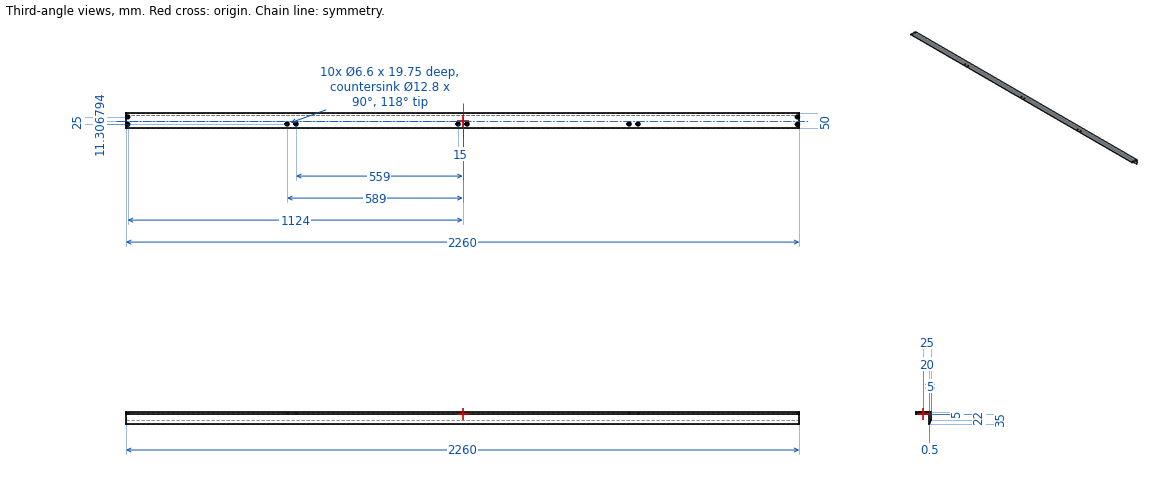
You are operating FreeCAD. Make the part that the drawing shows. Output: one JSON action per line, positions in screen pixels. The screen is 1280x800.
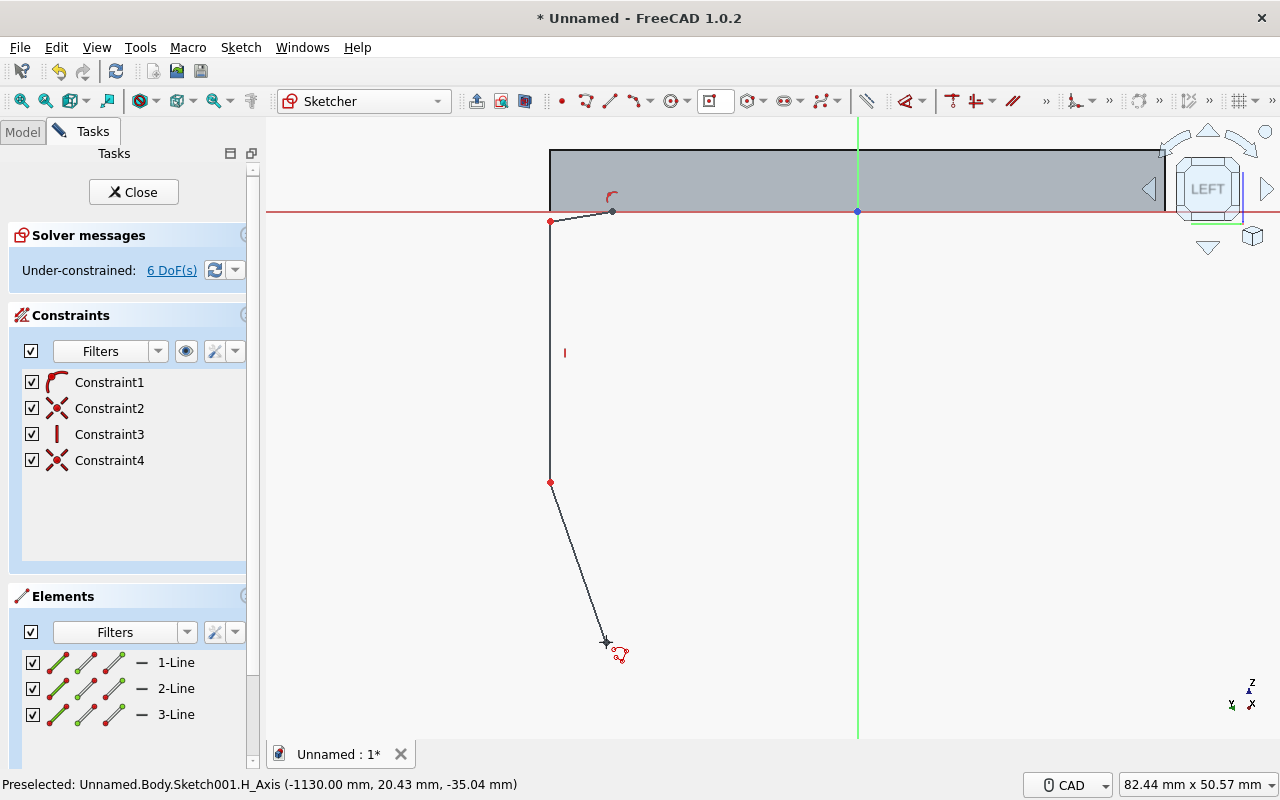
{"action": "scroll", "coordinate": [612, 642], "scroll_direction": "up", "scroll_amount": 5}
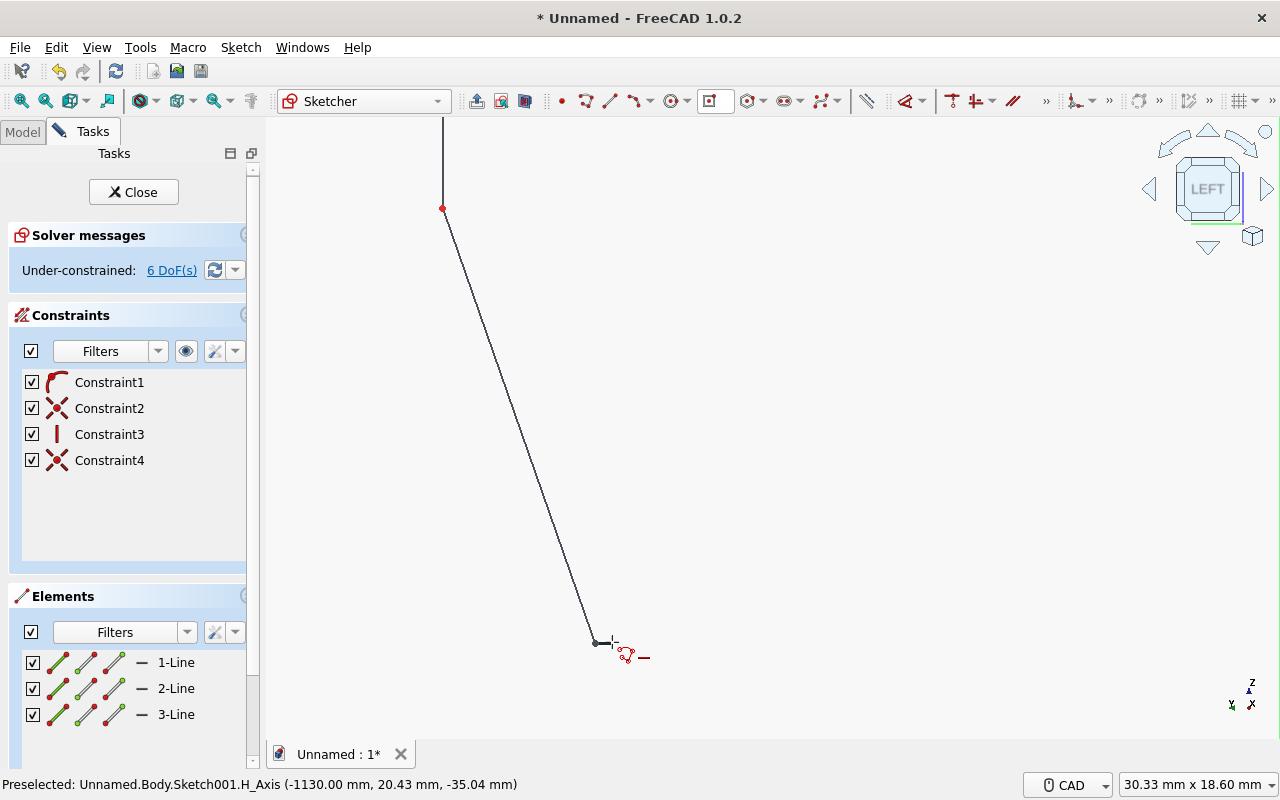
{"action": "left_click", "coordinate": [611, 641]}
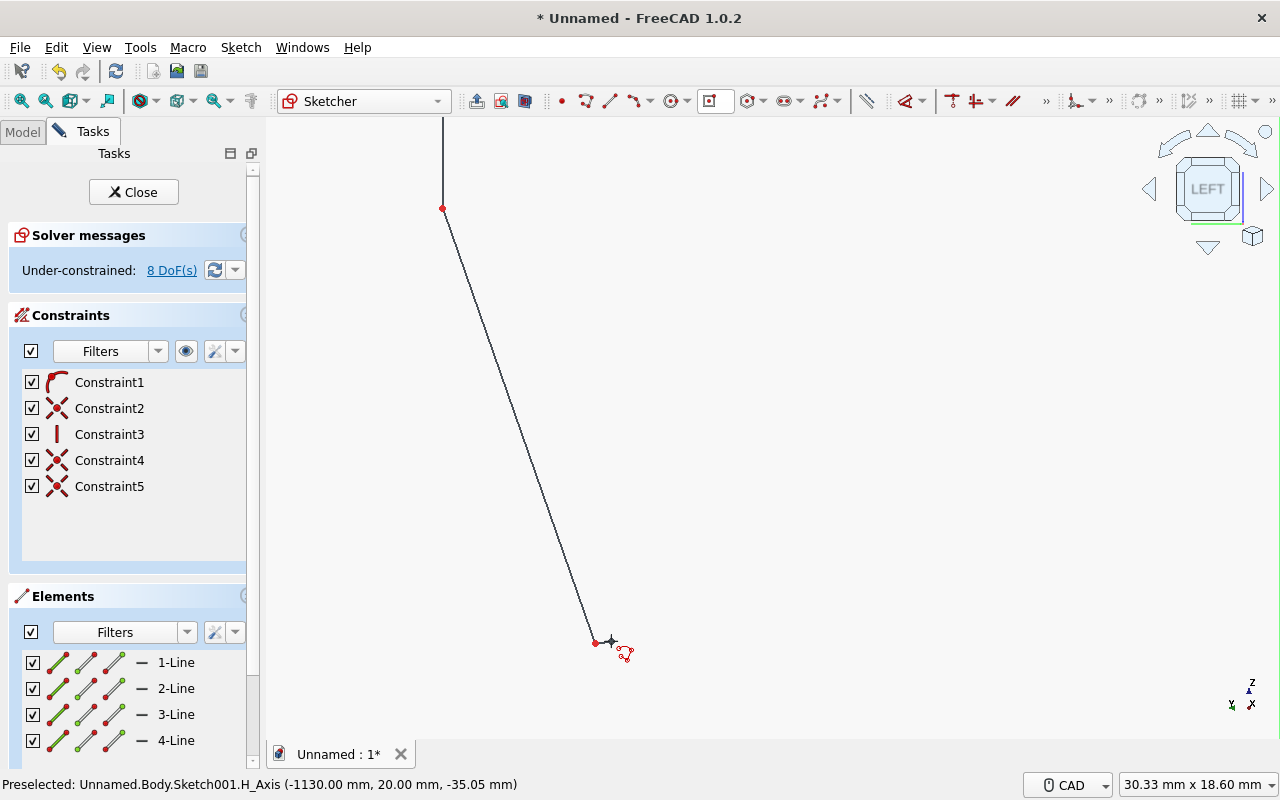
{"action": "scroll", "coordinate": [613, 644], "scroll_direction": "down", "scroll_amount": 5}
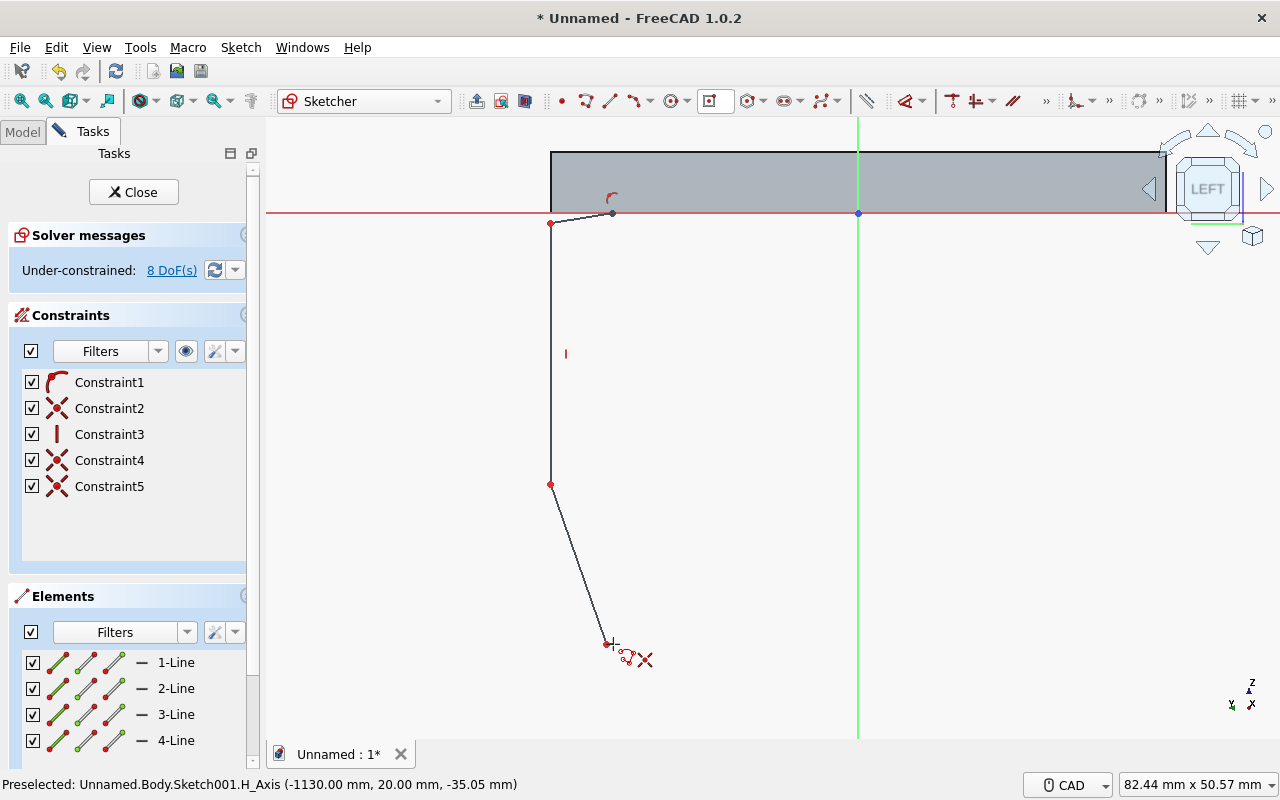
{"action": "left_click", "coordinate": [613, 213]}
{"action": "key", "text": "Escape"}
{"action": "key", "text": "Escape"}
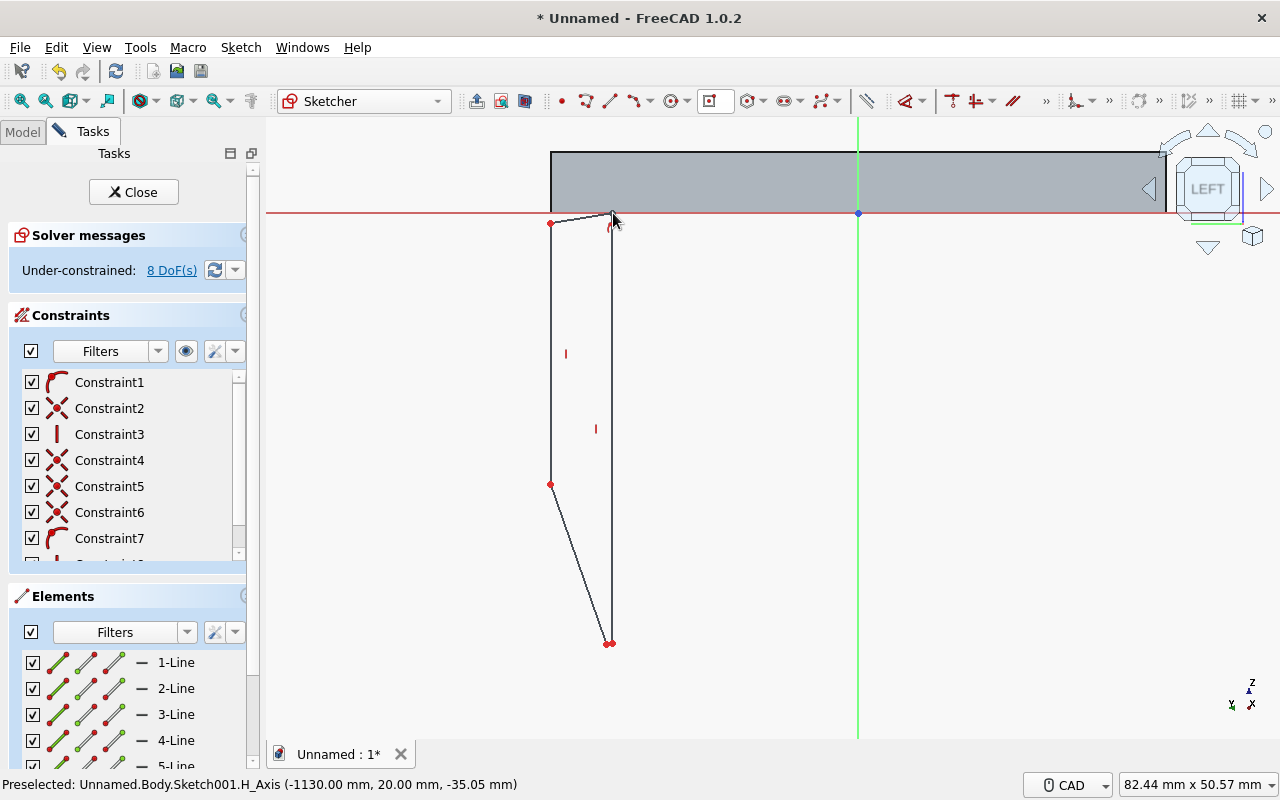
{"action": "left_click", "coordinate": [594, 216]}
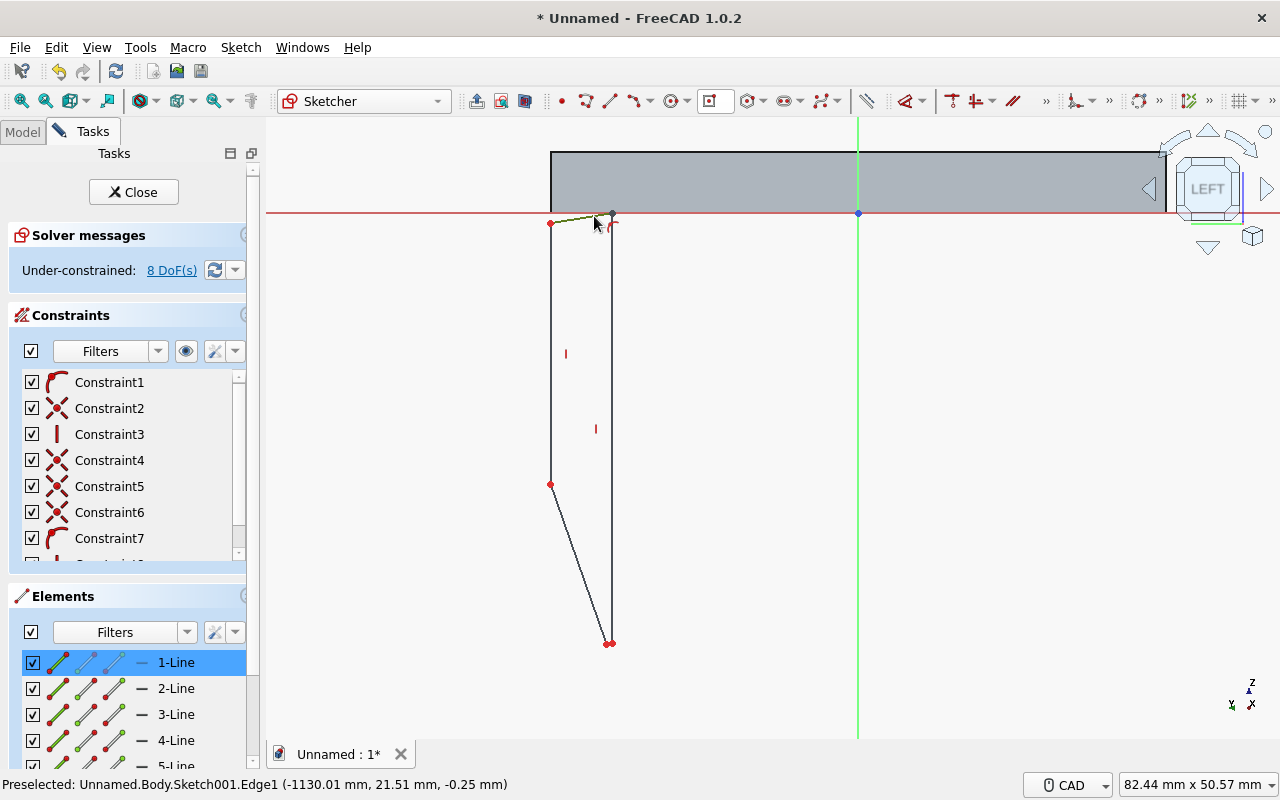
{"action": "left_click", "coordinate": [994, 102]}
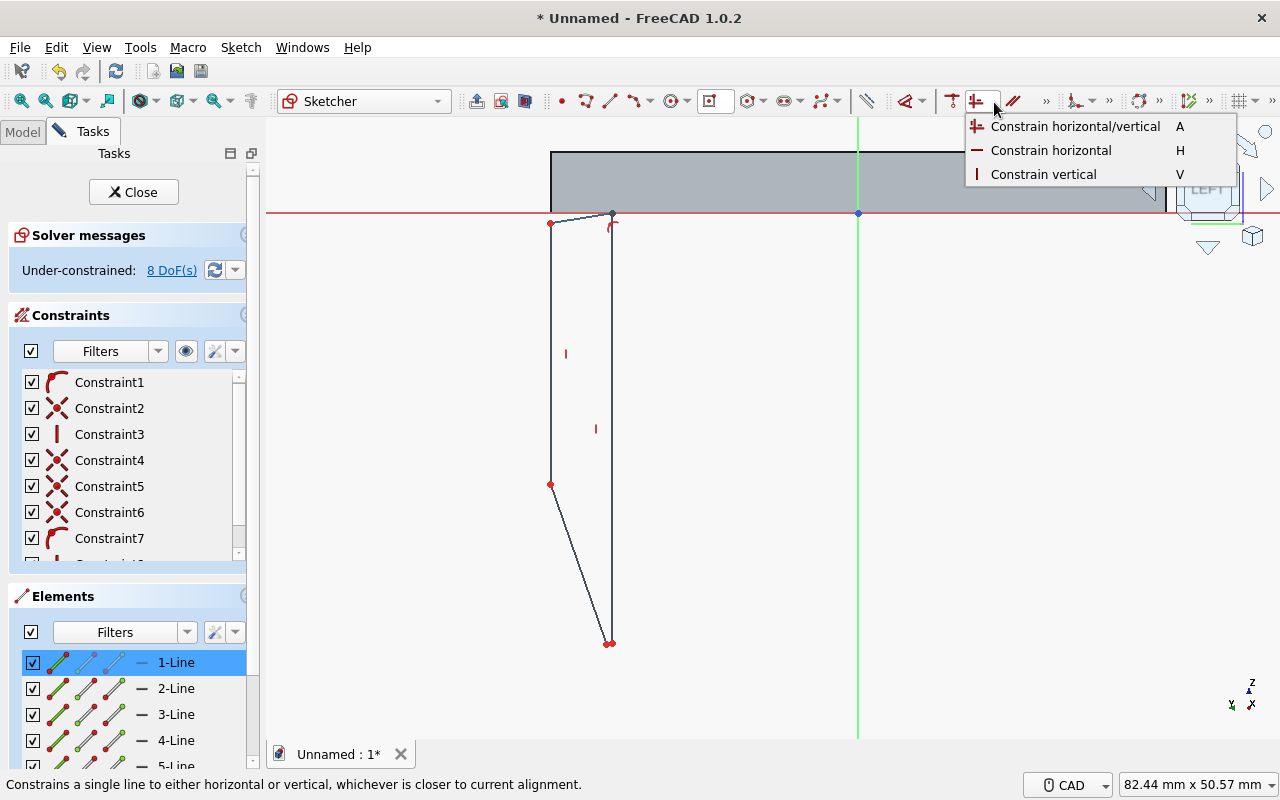
{"action": "left_click", "coordinate": [1101, 150]}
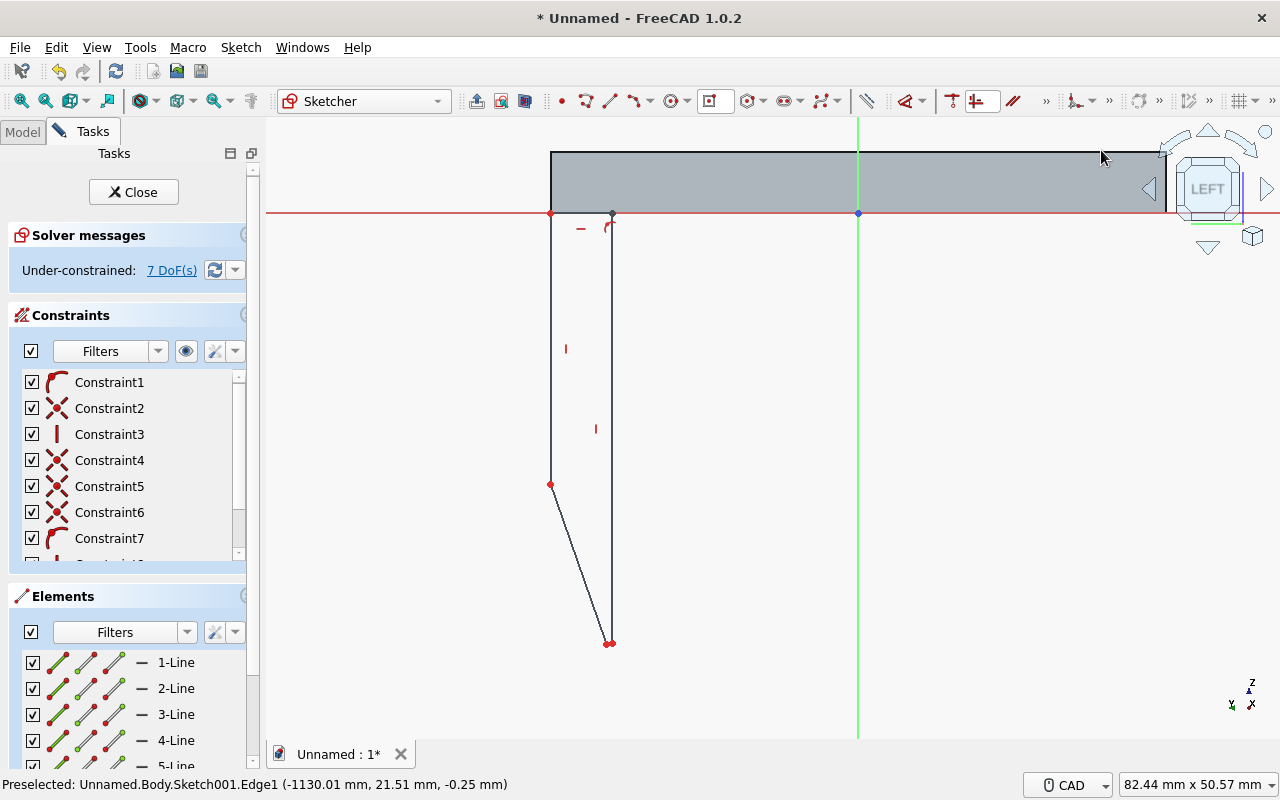
{"action": "scroll", "coordinate": [610, 644], "scroll_direction": "up", "scroll_amount": 8}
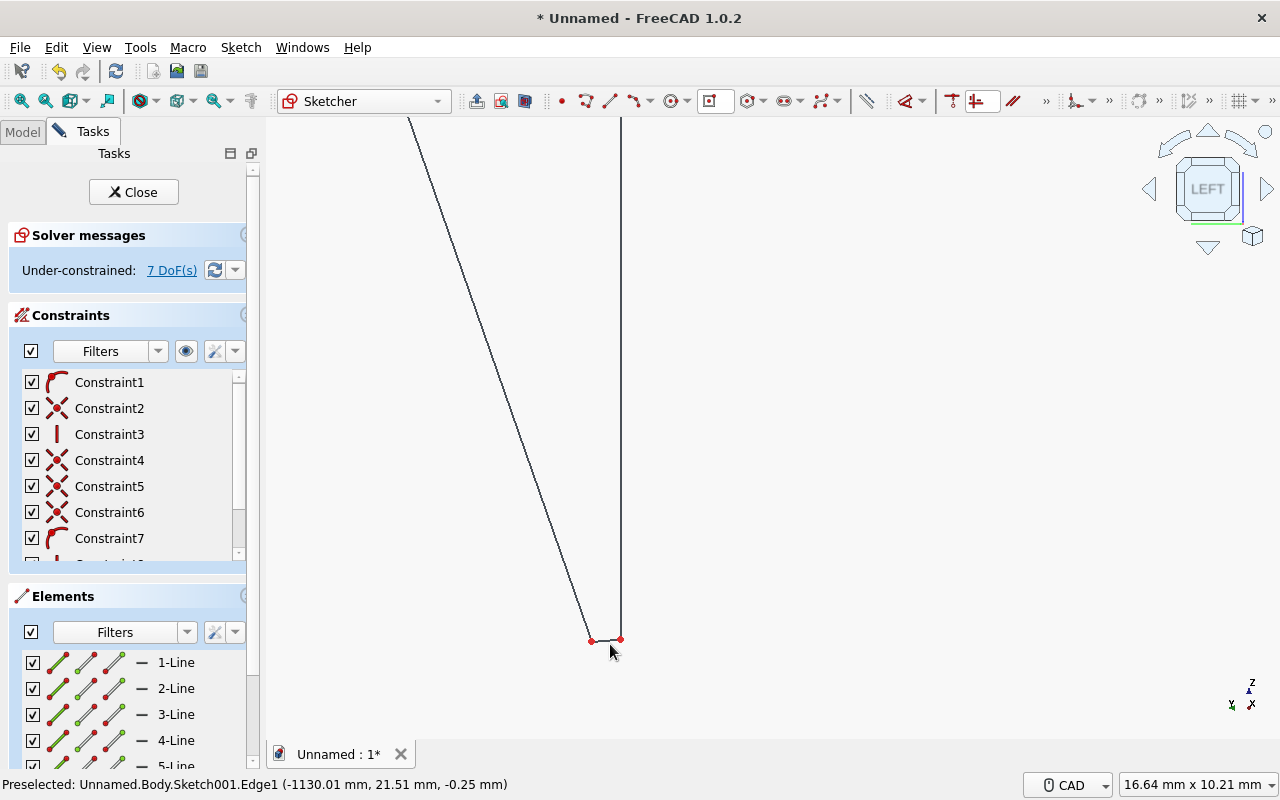
{"action": "left_click", "coordinate": [606, 641]}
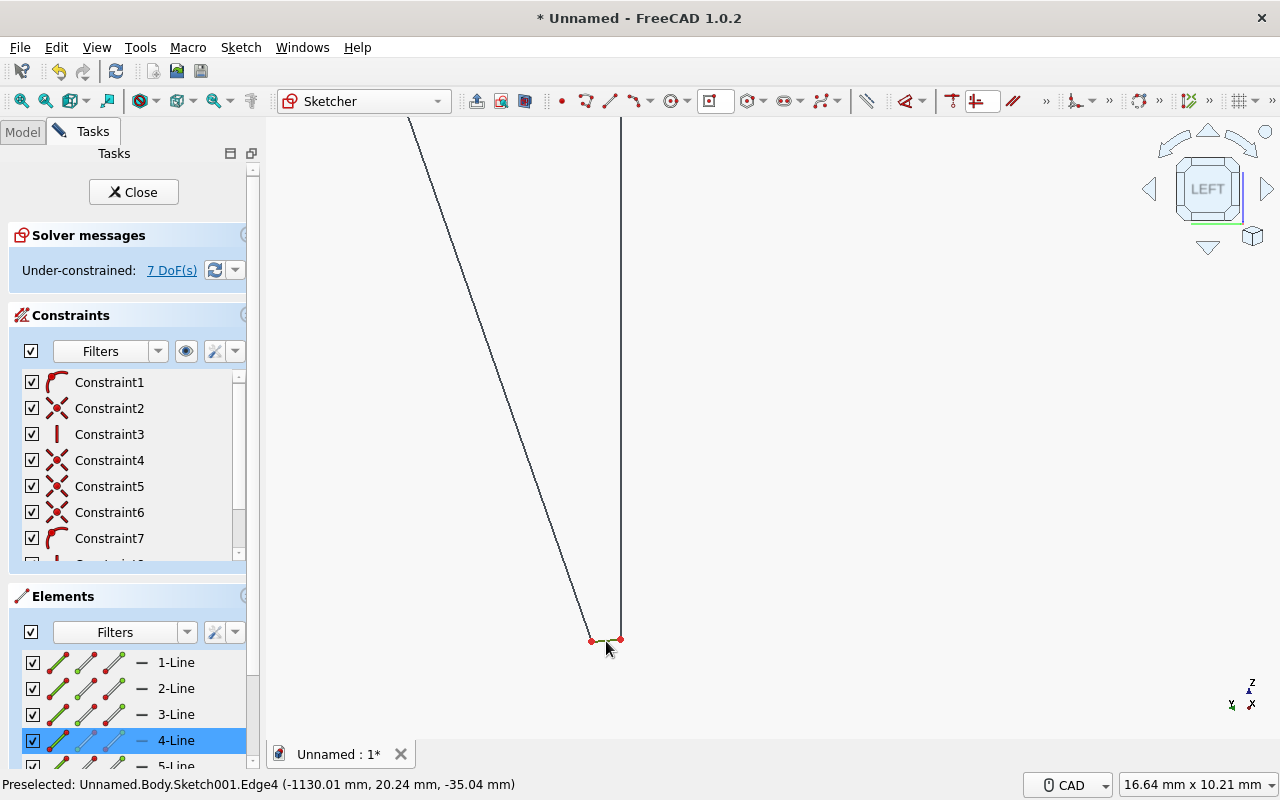
{"action": "key", "text": "h"}